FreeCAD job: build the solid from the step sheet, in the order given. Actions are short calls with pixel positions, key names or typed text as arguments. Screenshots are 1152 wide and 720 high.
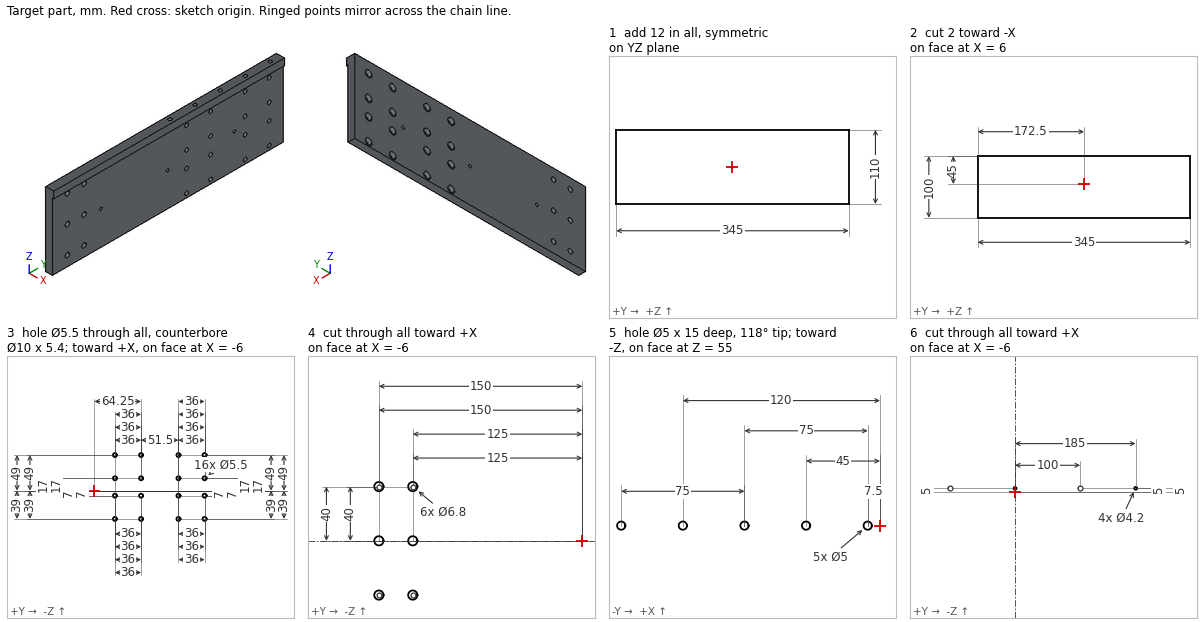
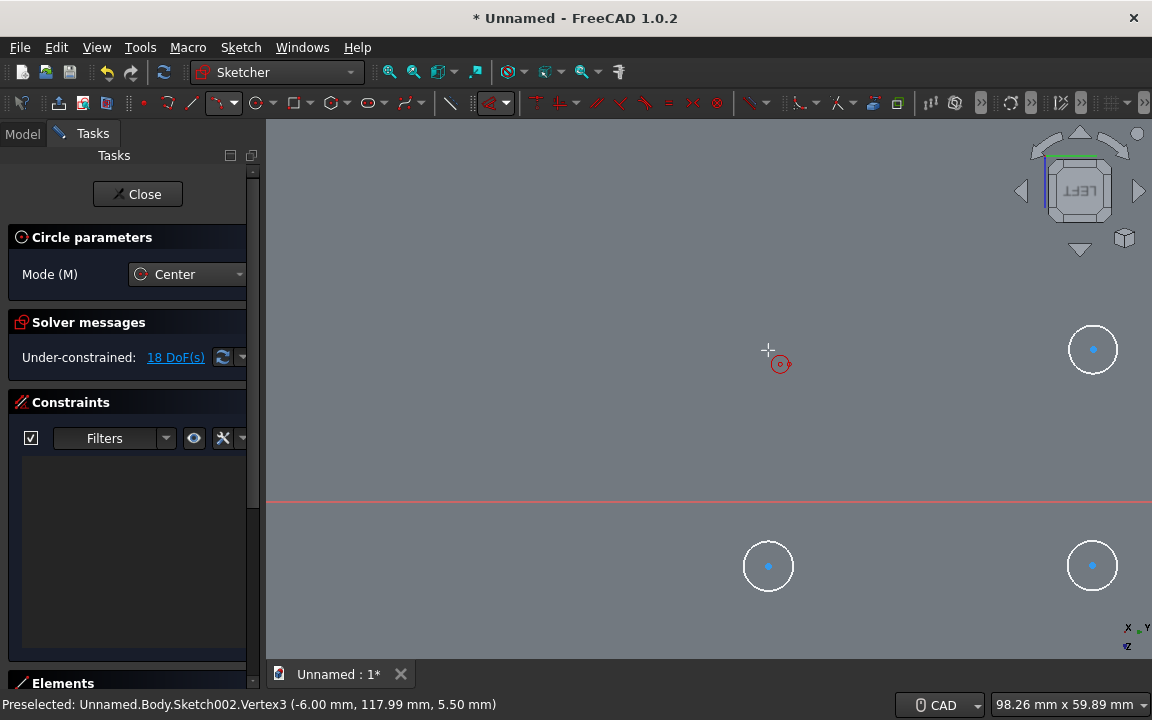
click(768, 349)
click(786, 331)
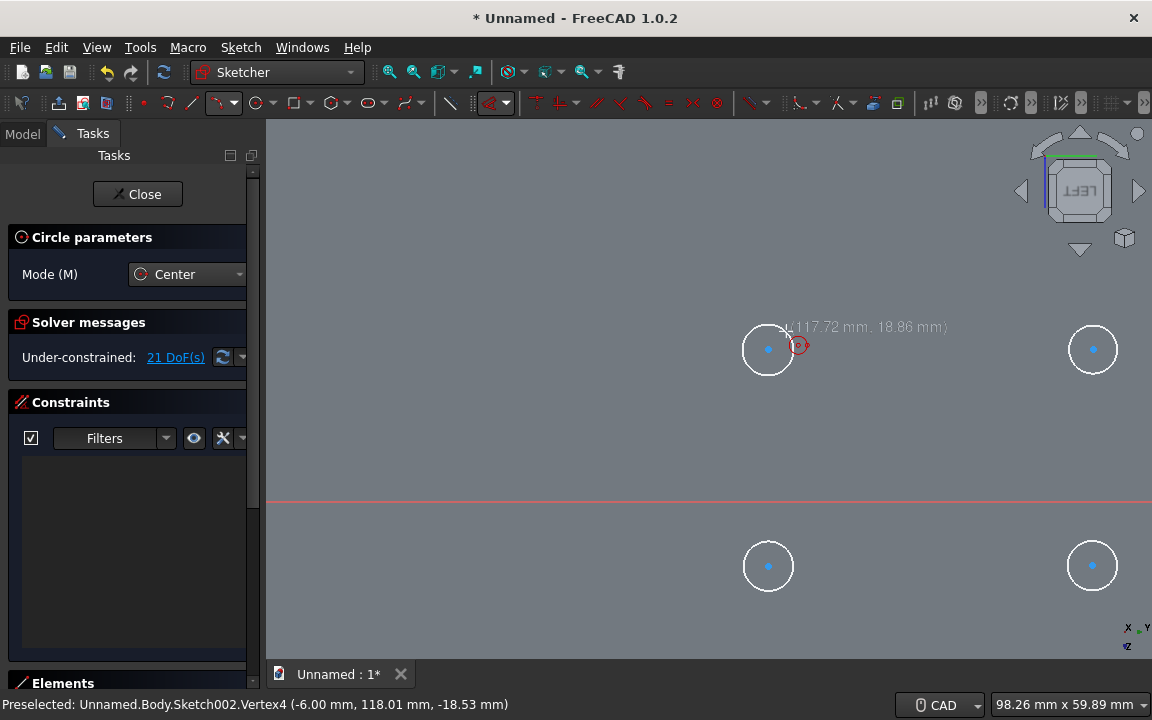
scroll(768, 349, down, 5)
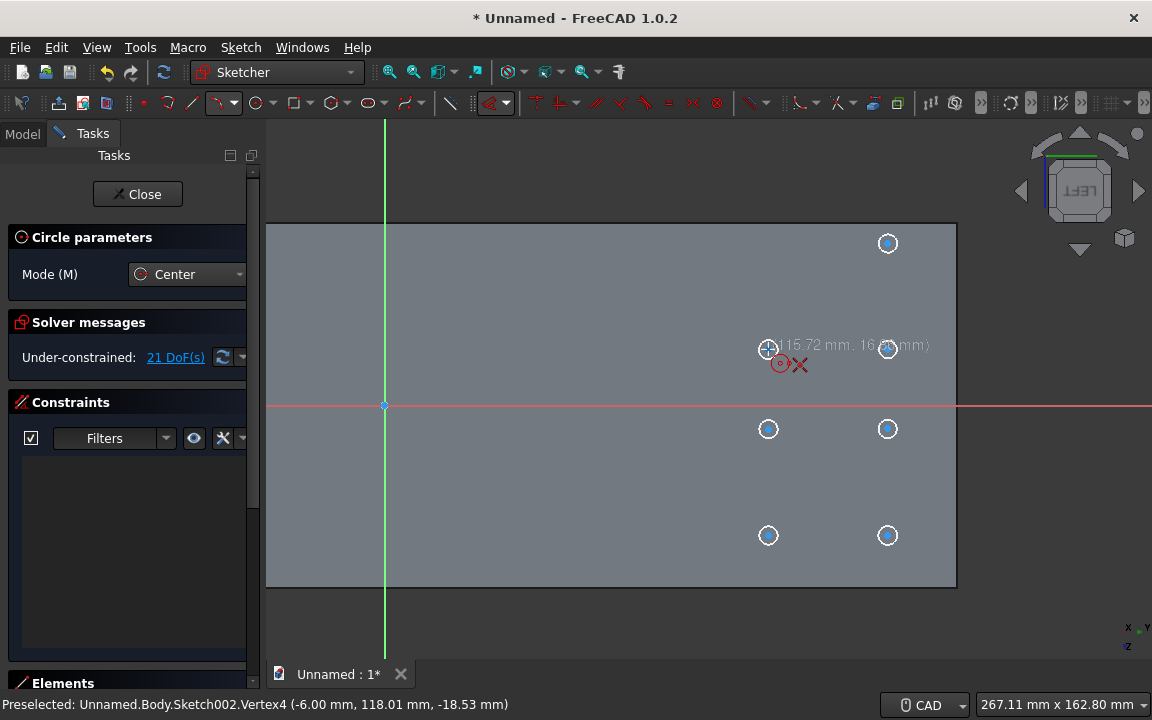
scroll(768, 243, up, 5)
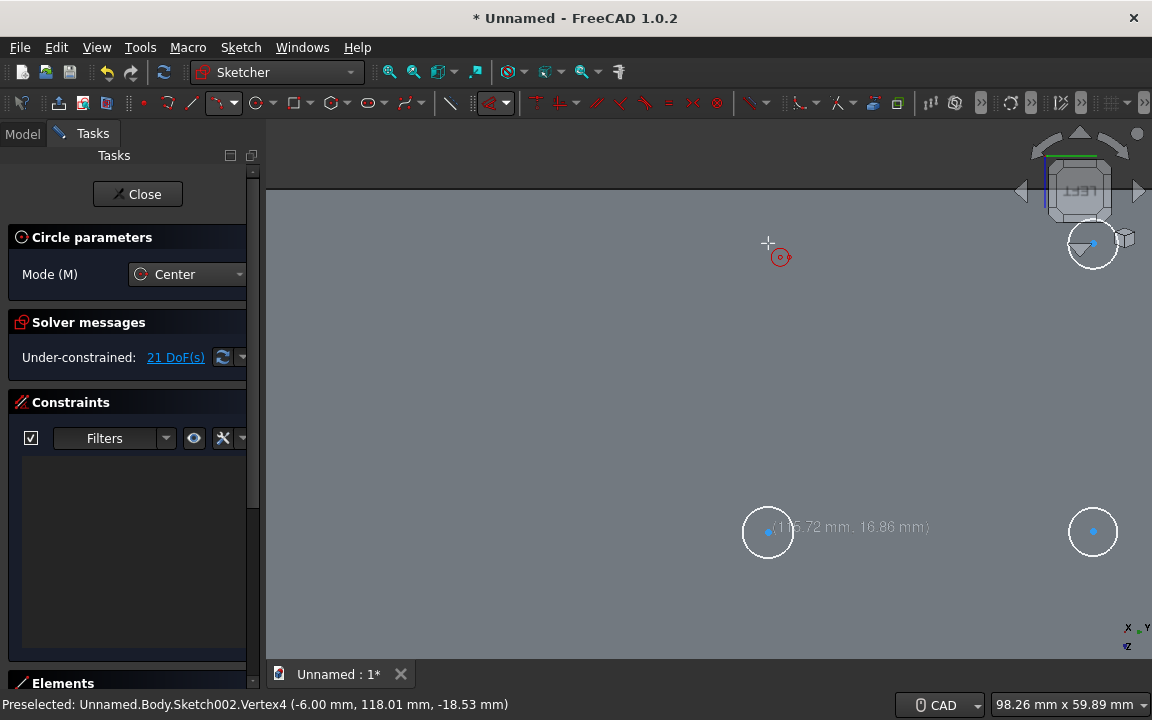
click(768, 243)
click(786, 225)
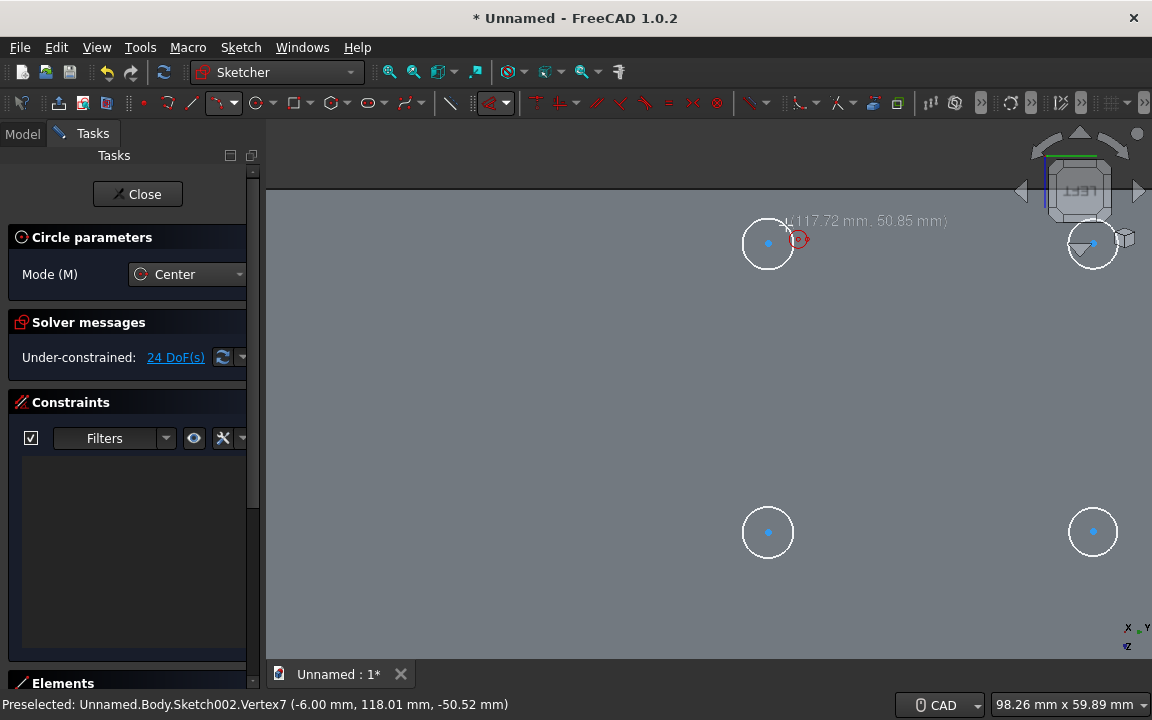
click(304, 243)
click(321, 225)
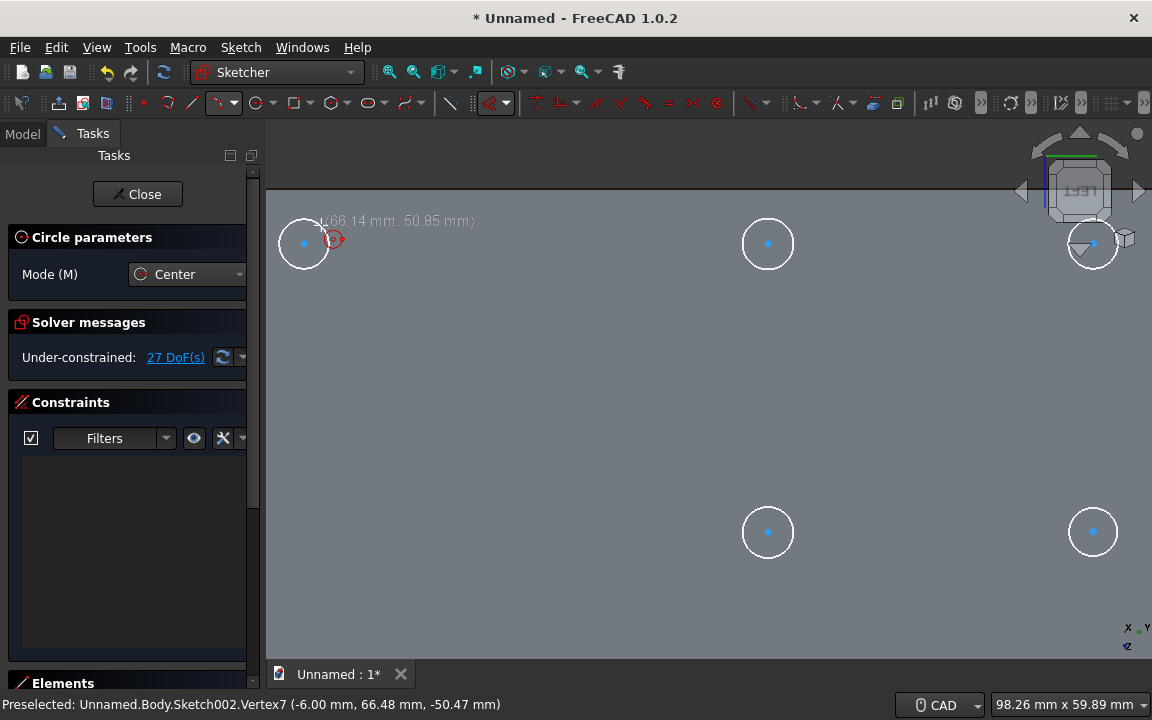
scroll(768, 243, down, 5)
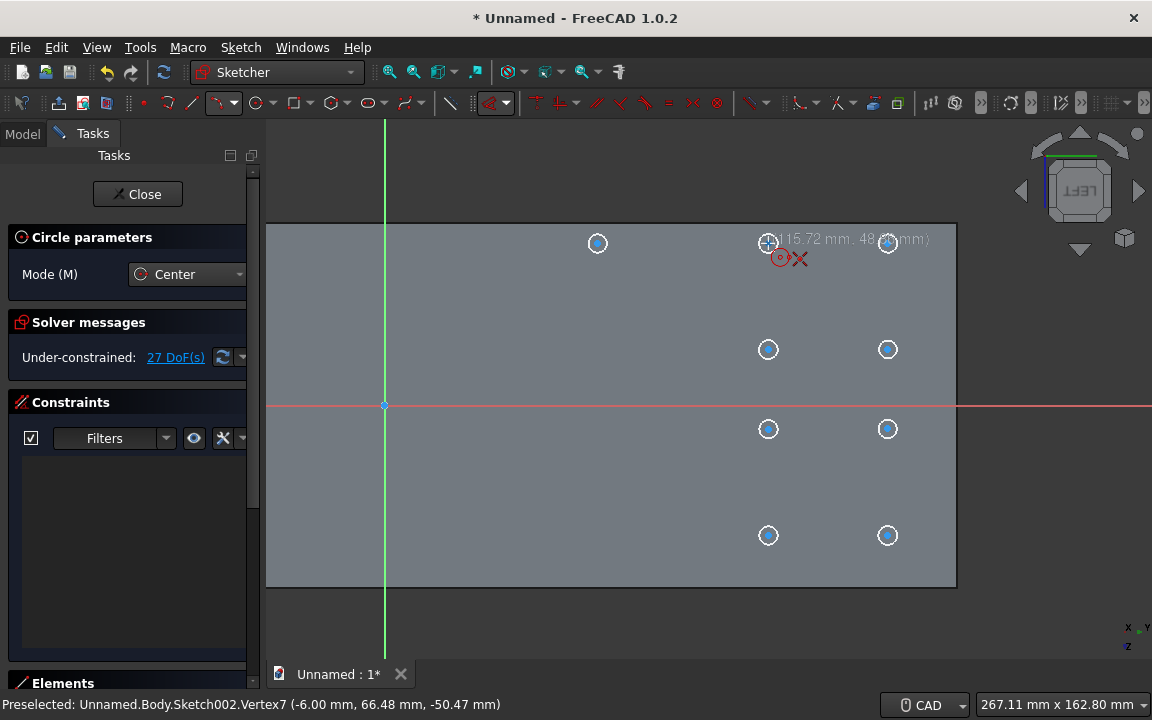
scroll(478, 243, up, 5)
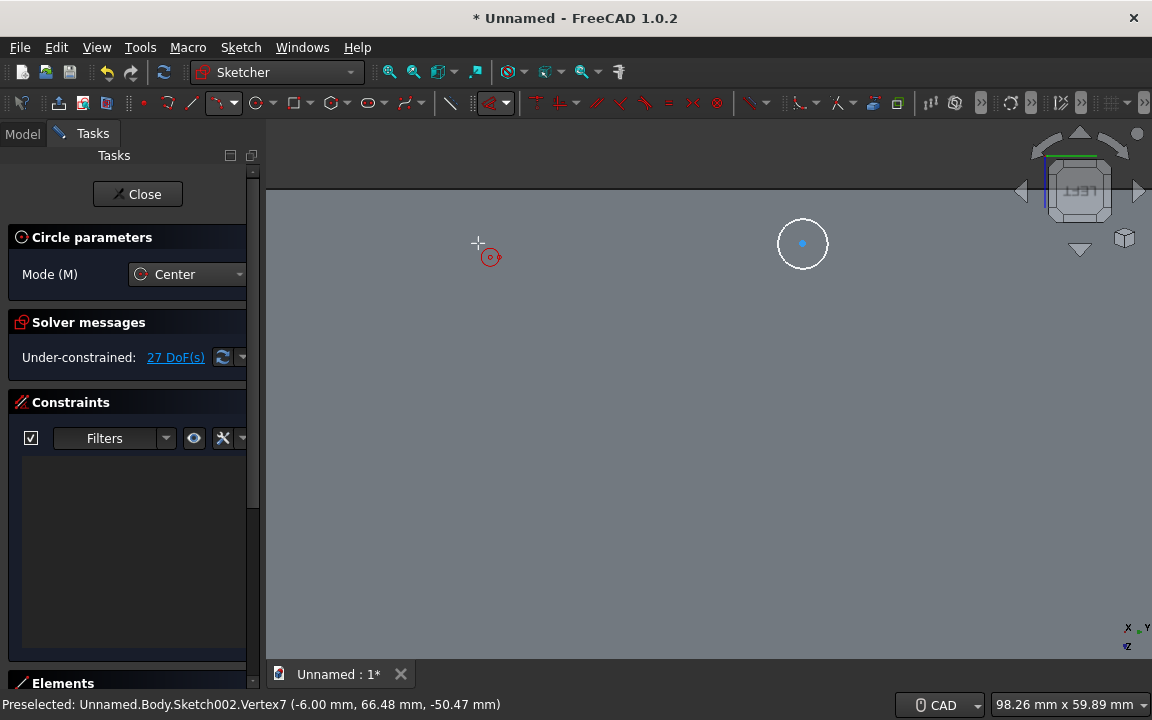
click(478, 243)
click(496, 225)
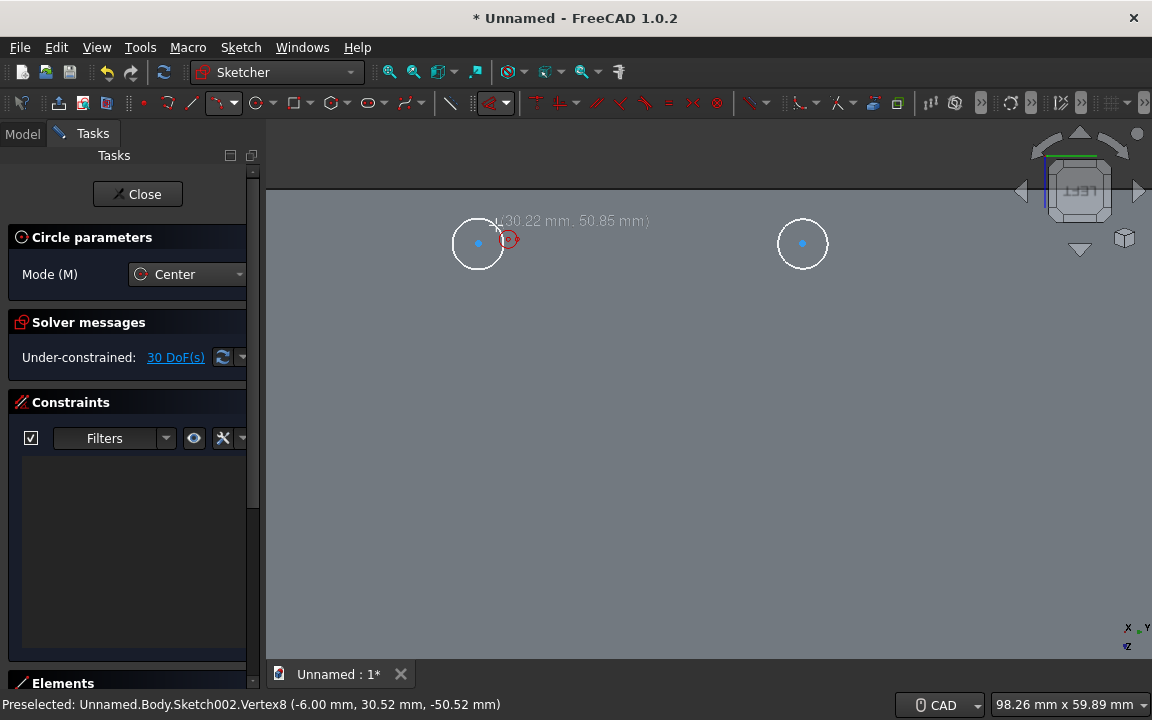
click(803, 531)
click(820, 514)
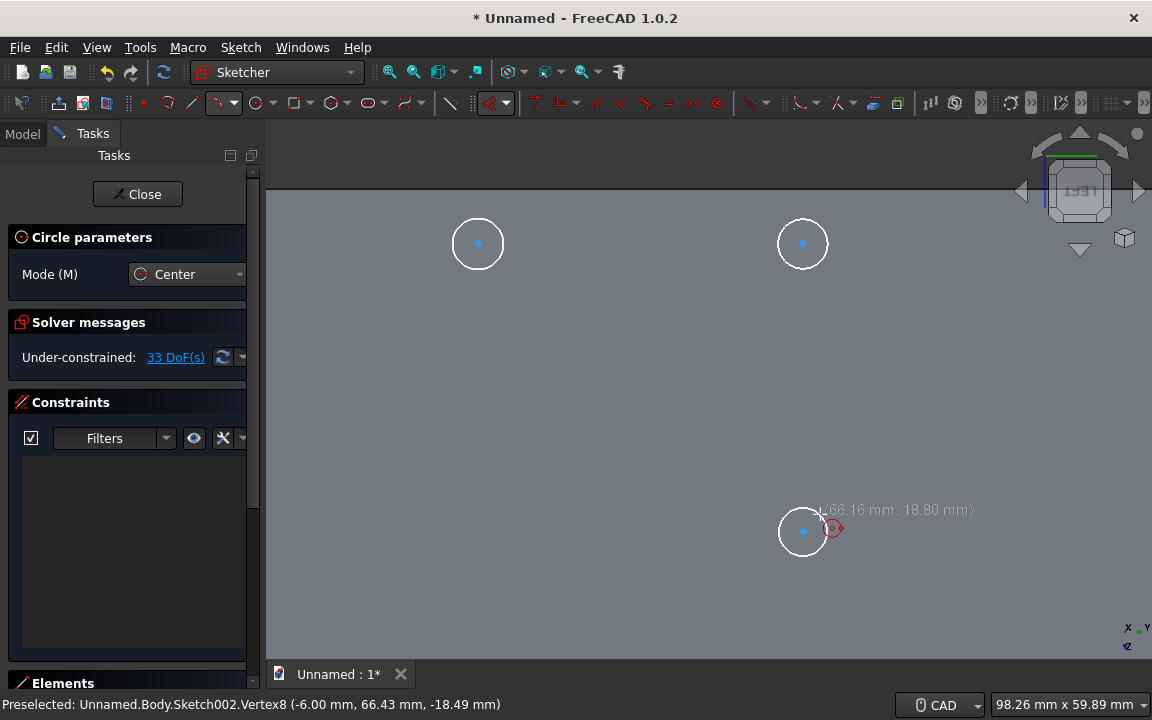
click(478, 531)
click(496, 514)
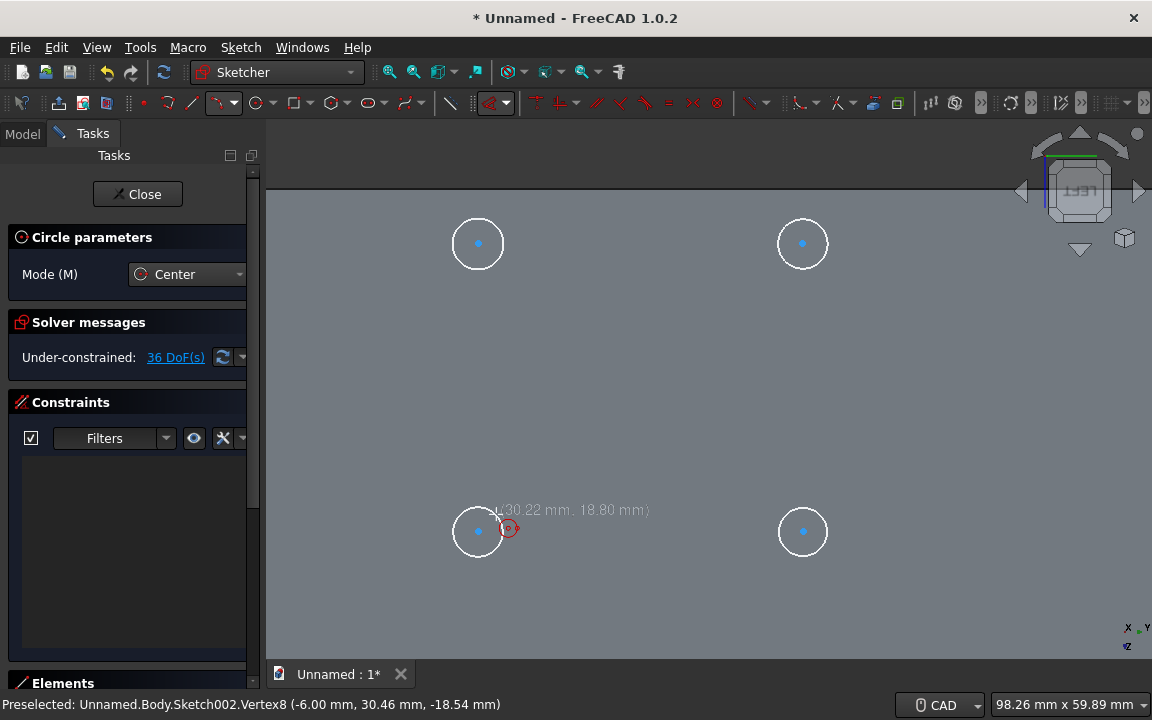
scroll(478, 243, down, 5)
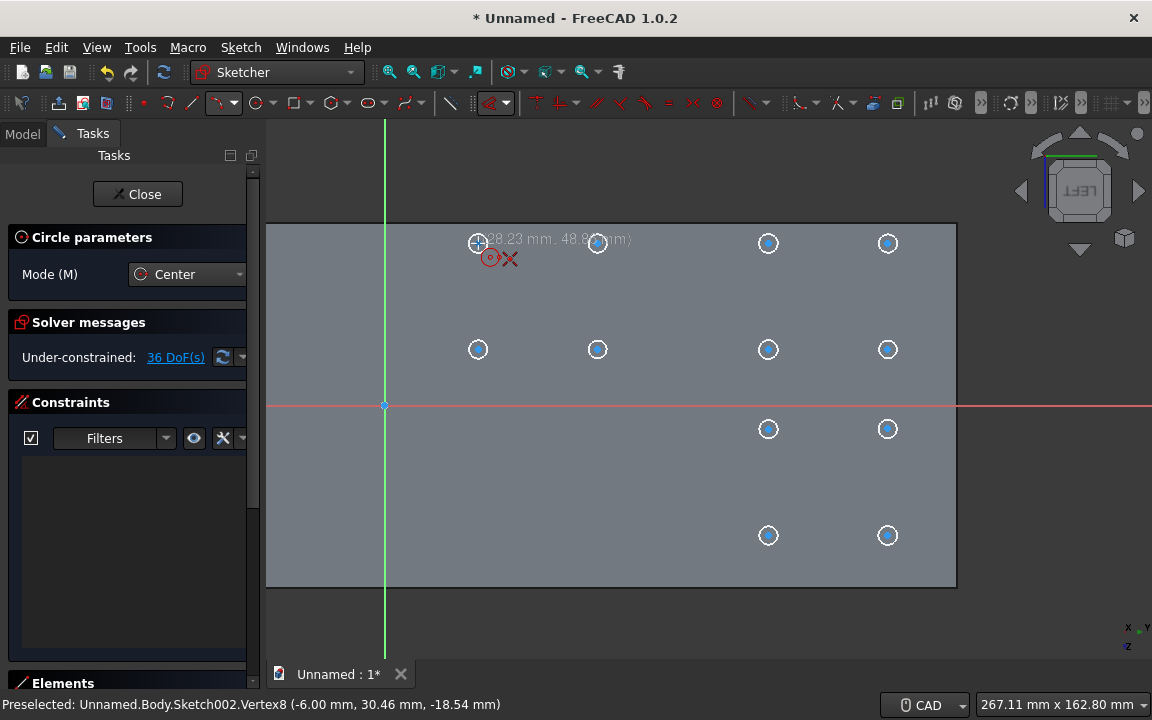
scroll(598, 429, up, 5)